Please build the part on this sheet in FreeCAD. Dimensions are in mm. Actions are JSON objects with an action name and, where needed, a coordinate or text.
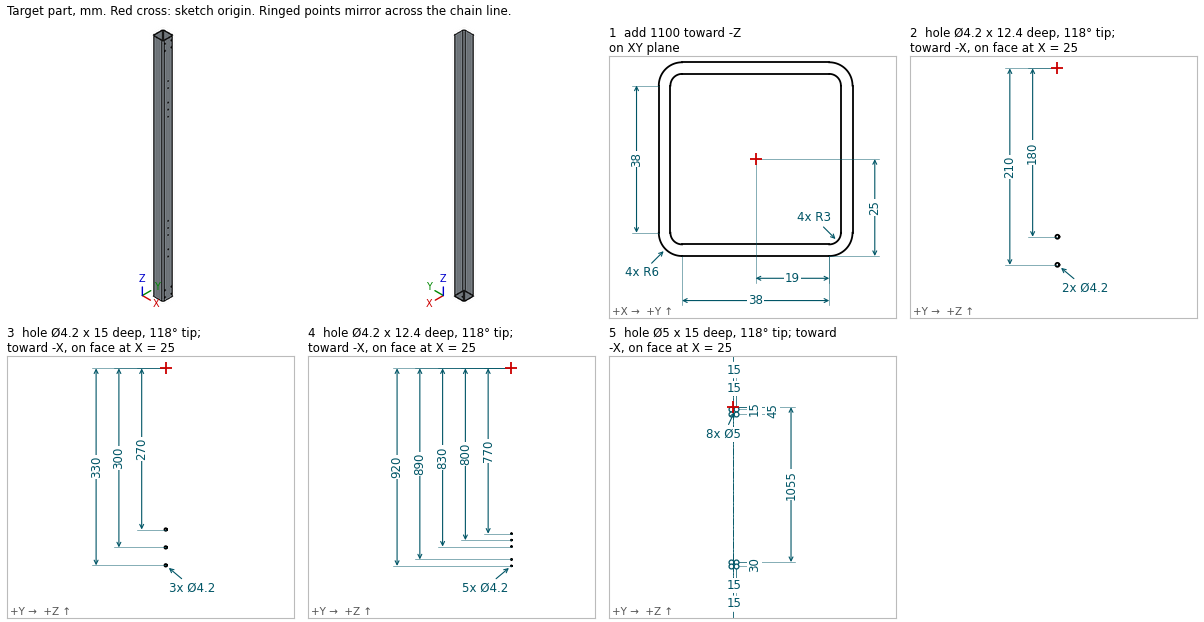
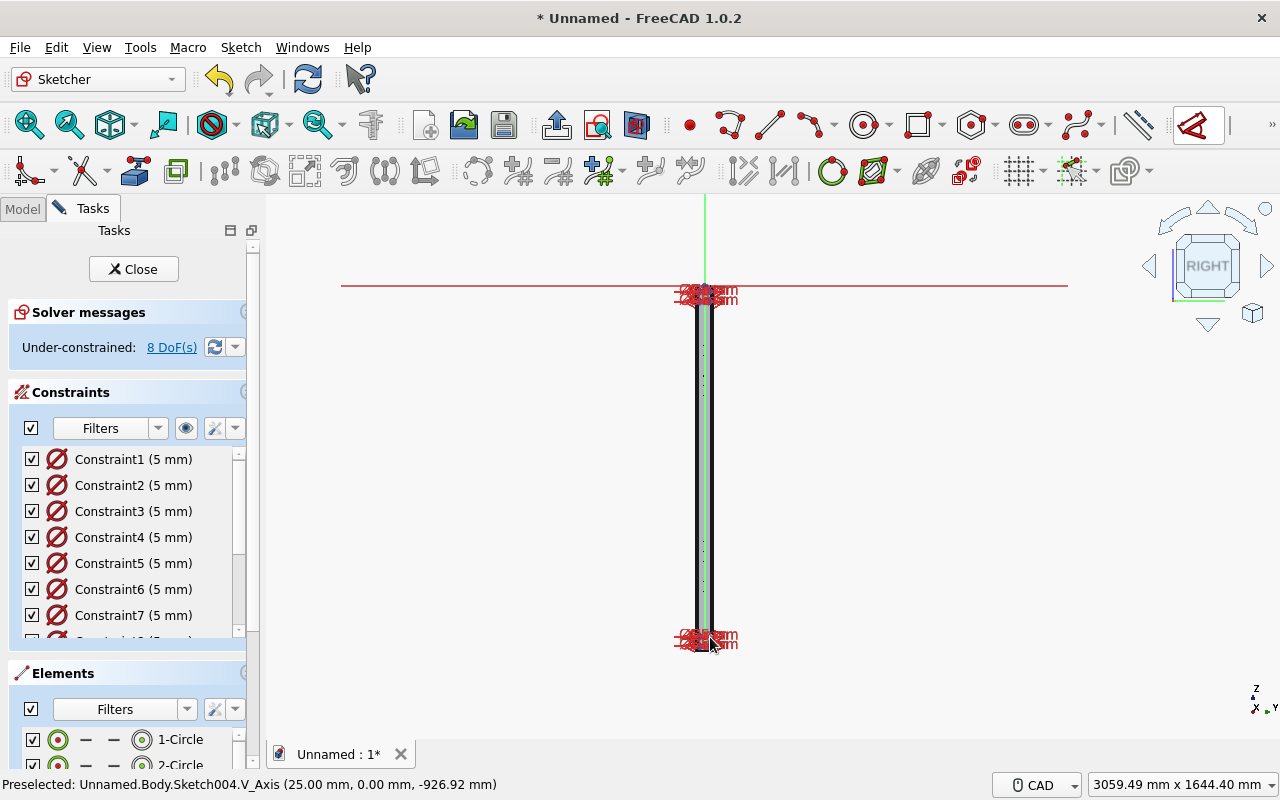
{"action": "scroll", "coordinate": [710, 292], "scroll_direction": "up", "scroll_amount": 11}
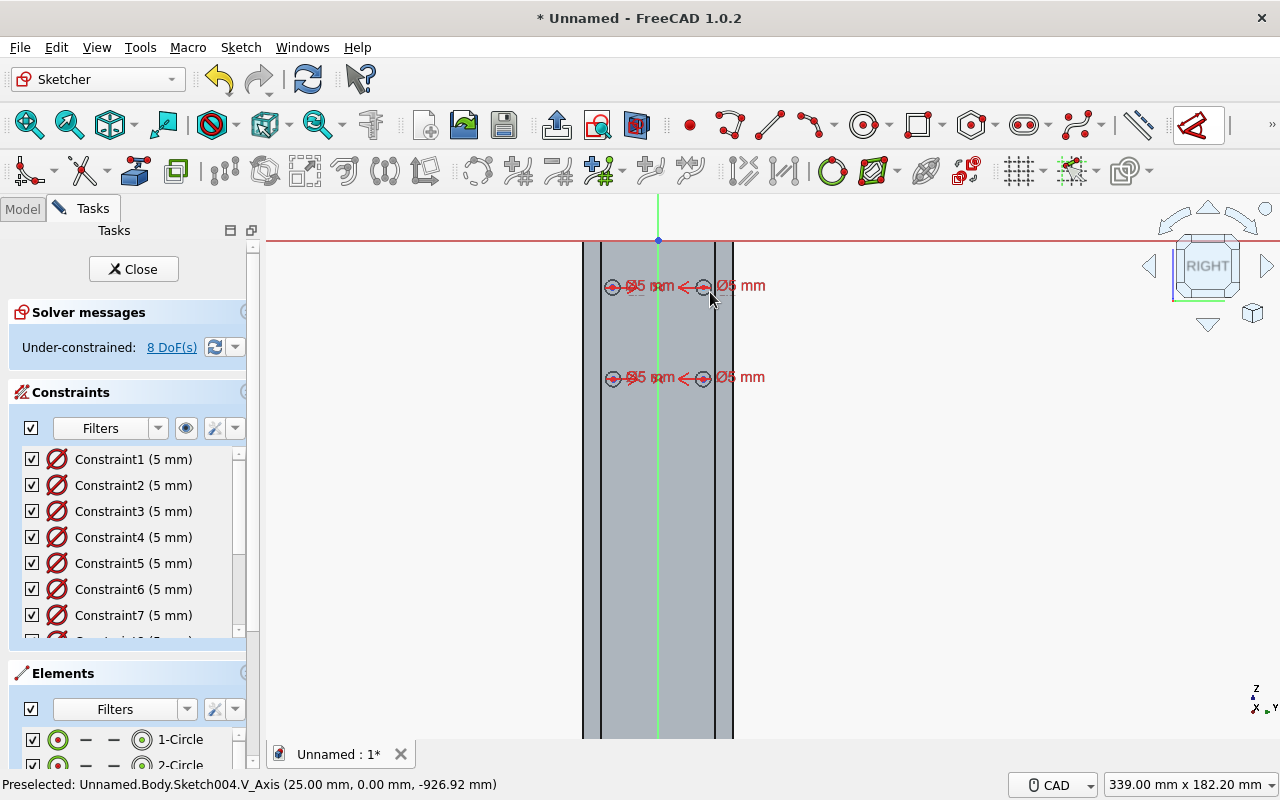
{"action": "left_click", "coordinate": [704, 288]}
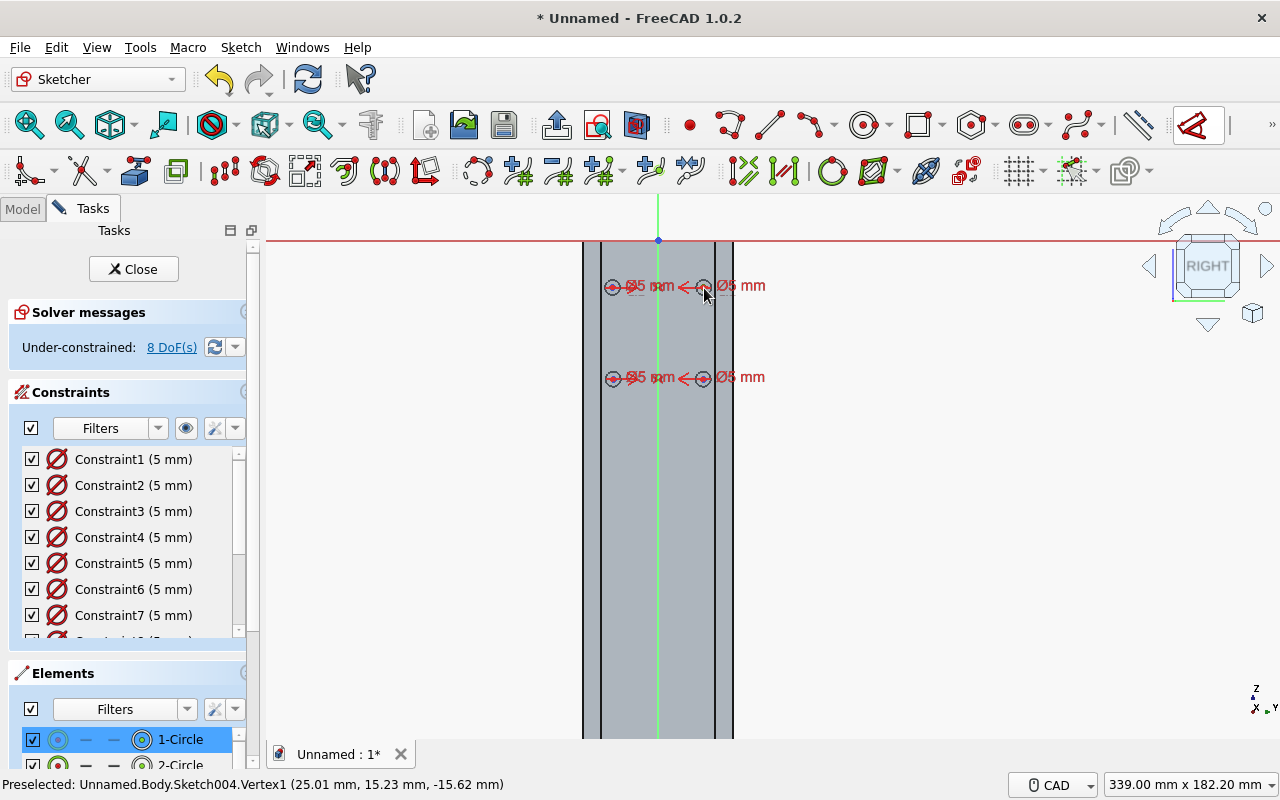
{"action": "left_click", "coordinate": [1218, 126]}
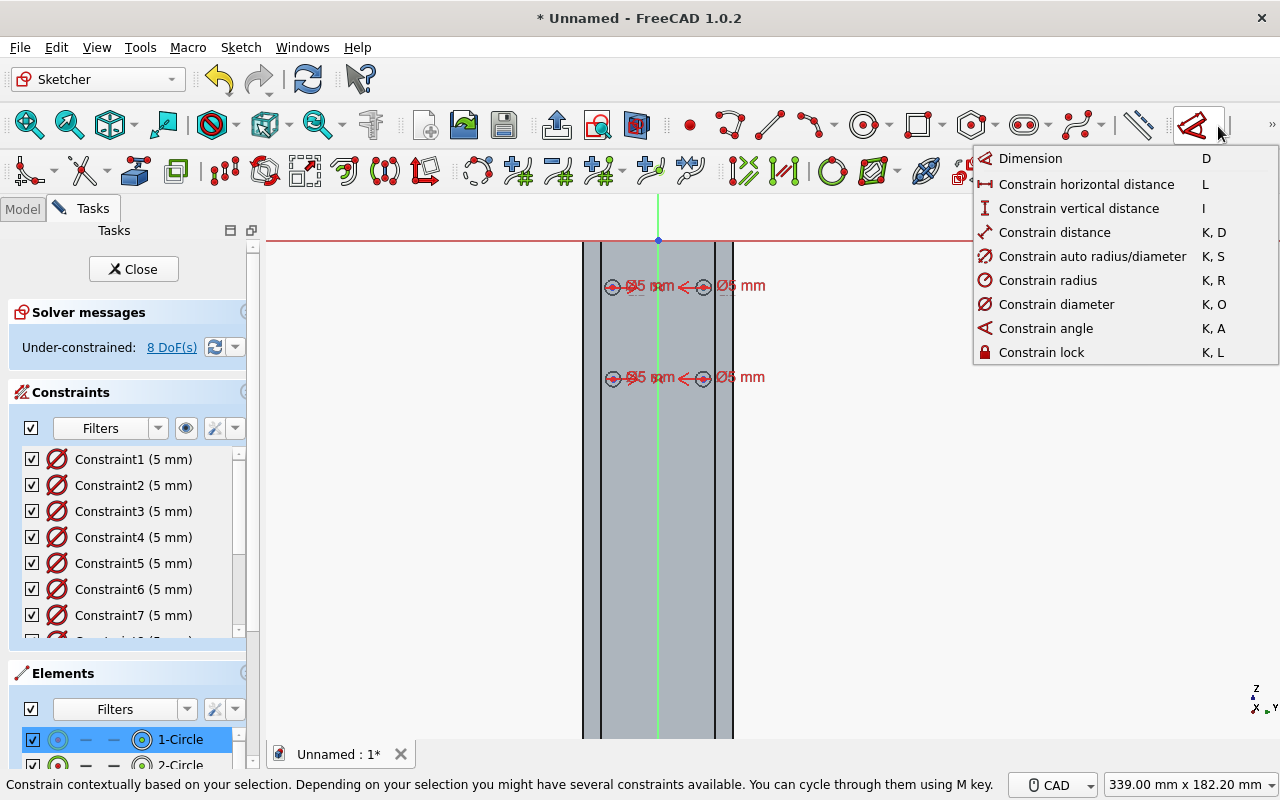
{"action": "left_click", "coordinate": [1126, 184]}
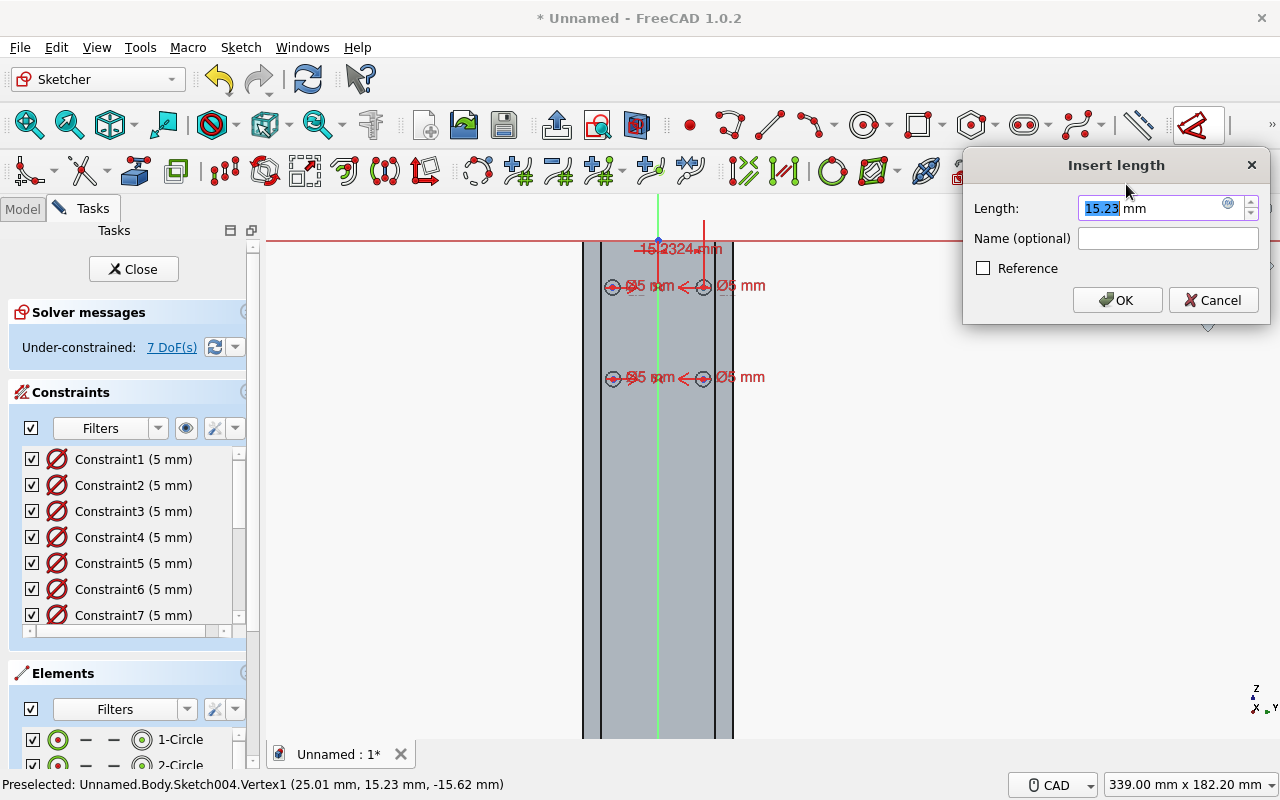
{"action": "type", "text": "15"}
{"action": "key", "text": "Return"}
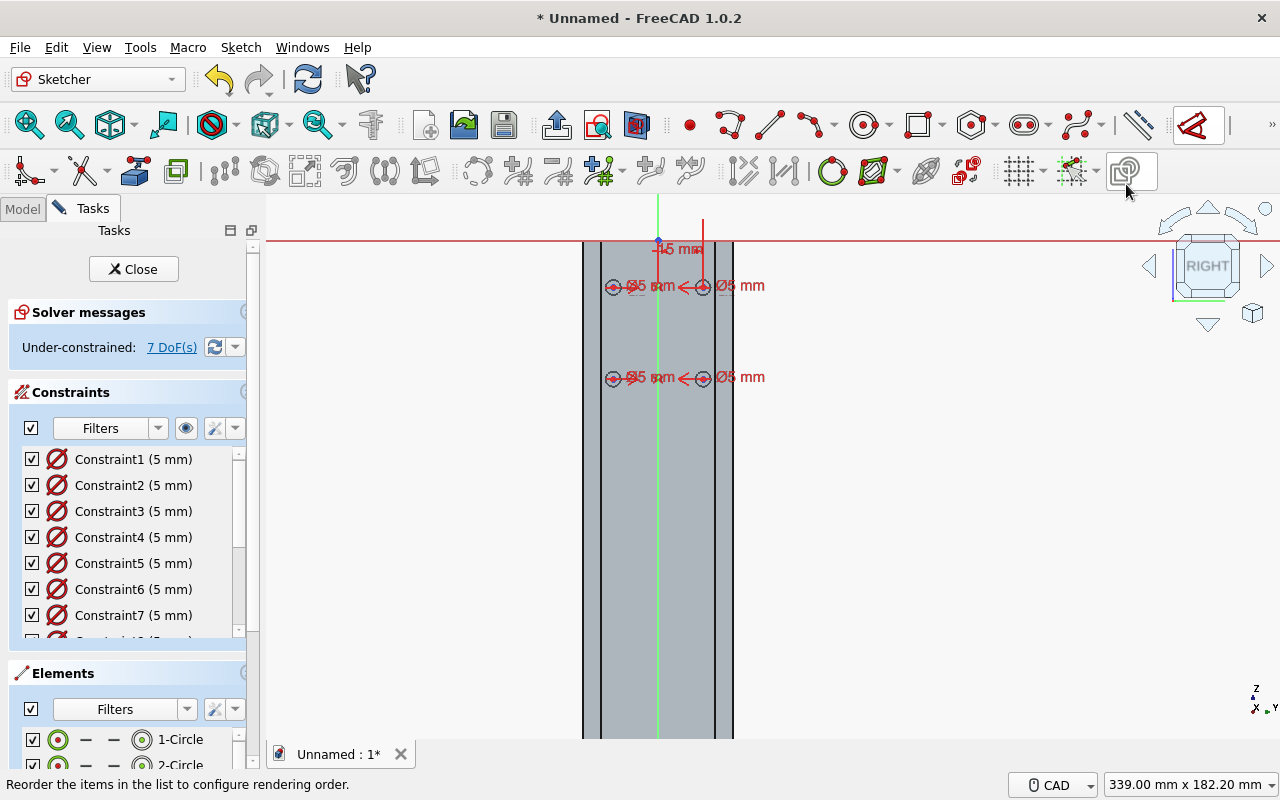
{"action": "left_click", "coordinate": [703, 288]}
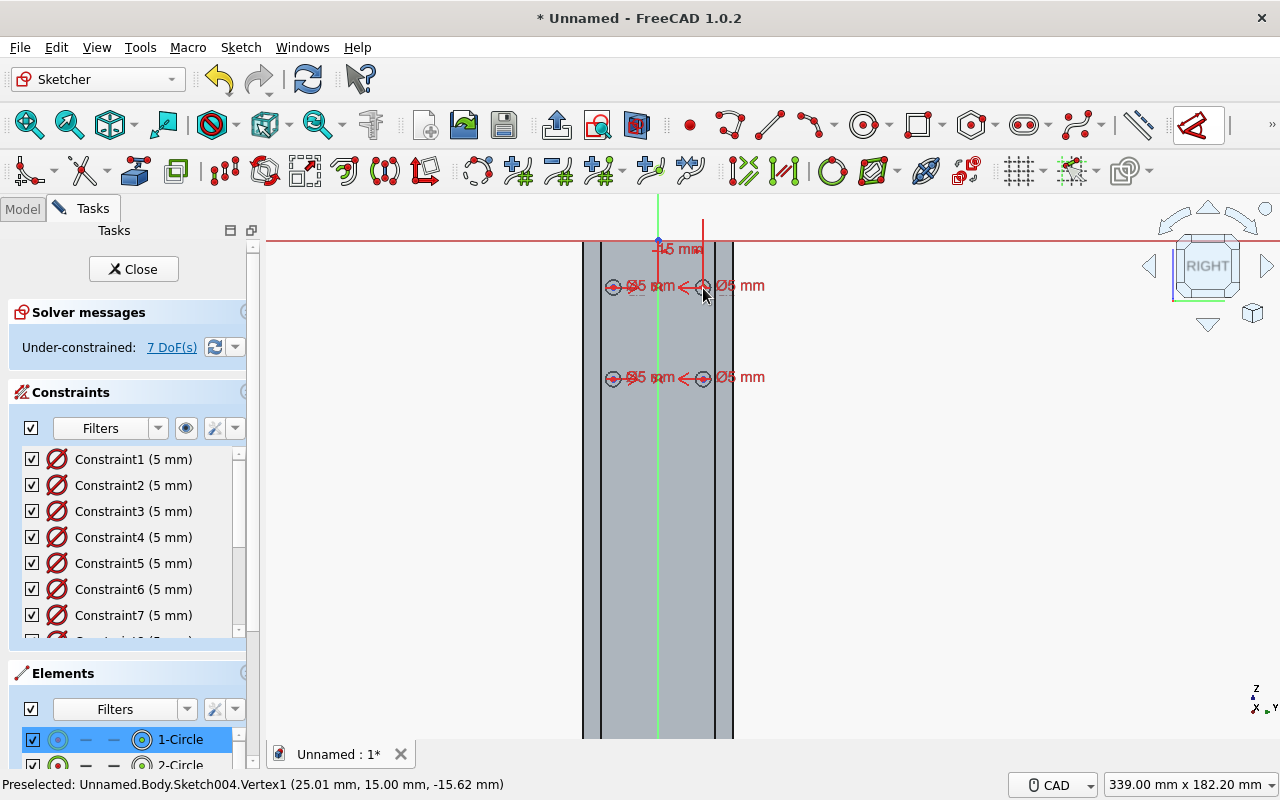
{"action": "left_click", "coordinate": [1218, 126]}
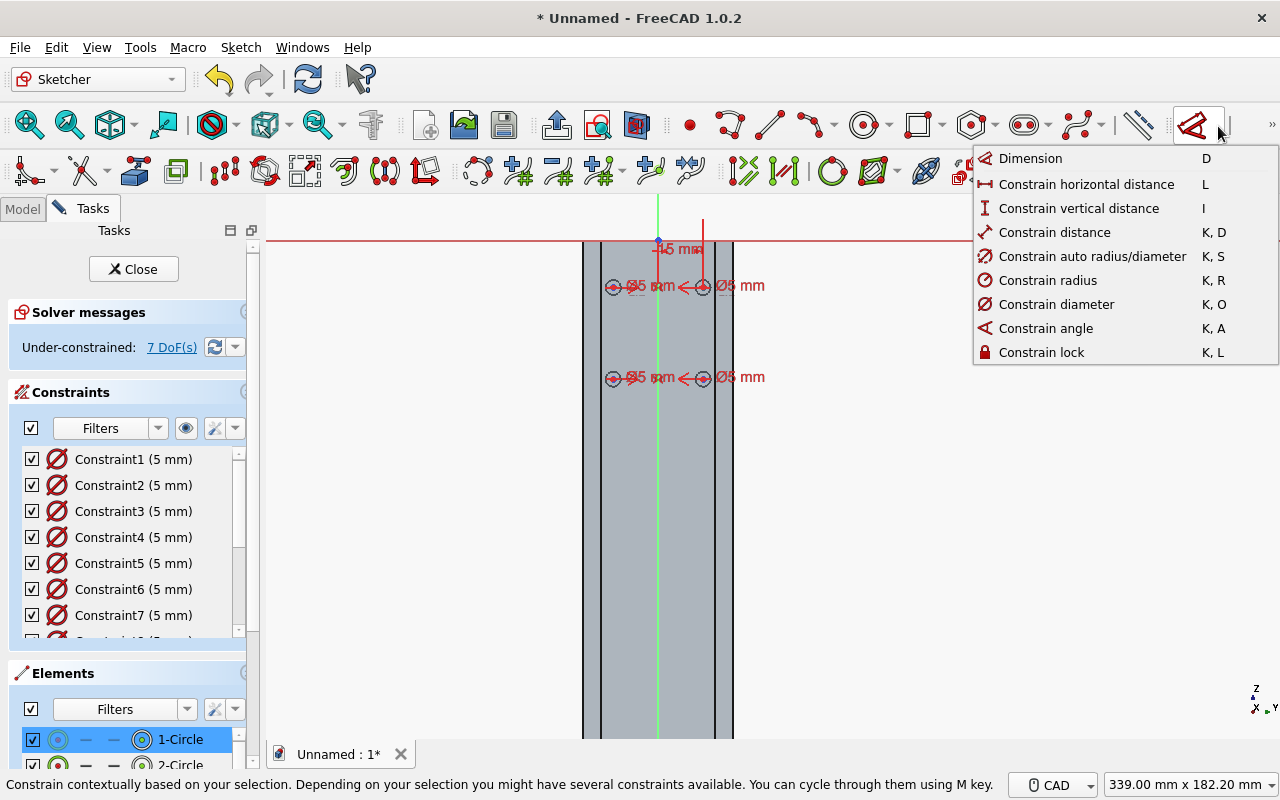
{"action": "left_click", "coordinate": [1126, 208]}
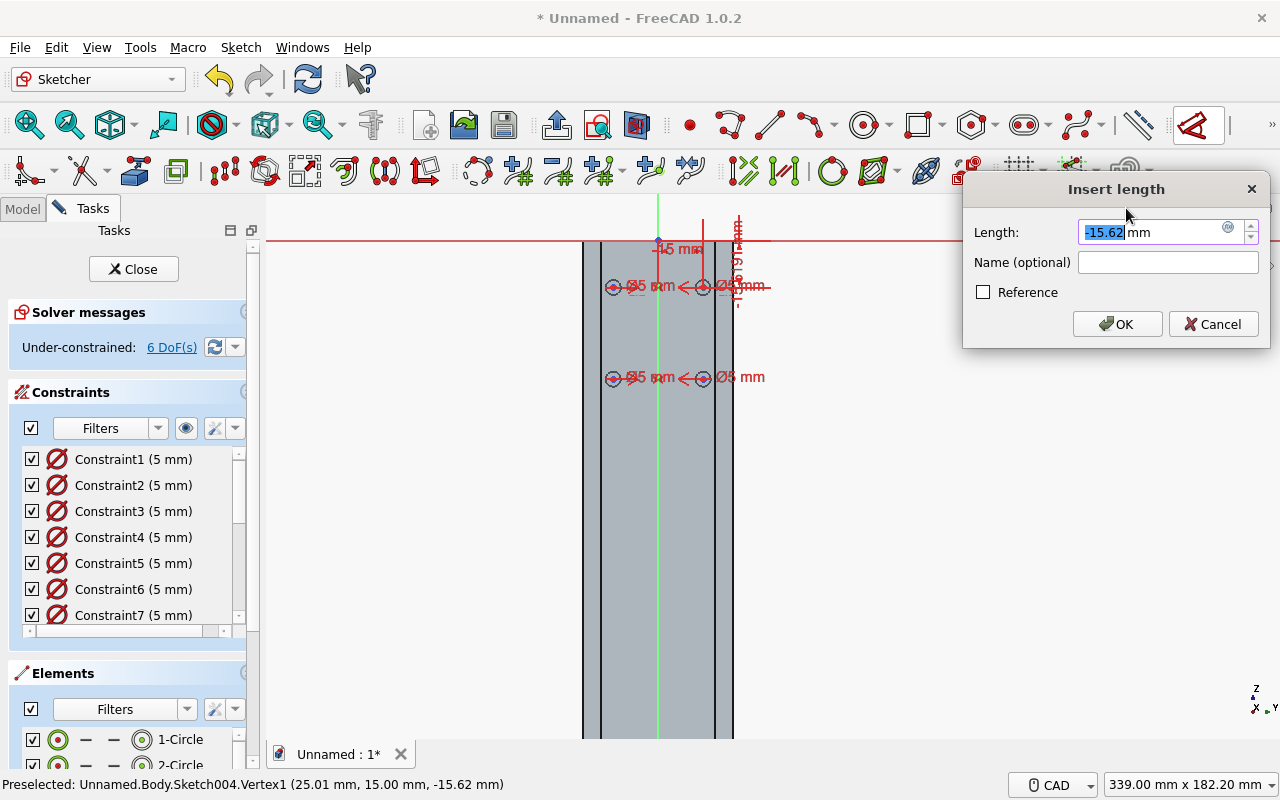
{"action": "type", "text": "-15"}
{"action": "key", "text": "Return"}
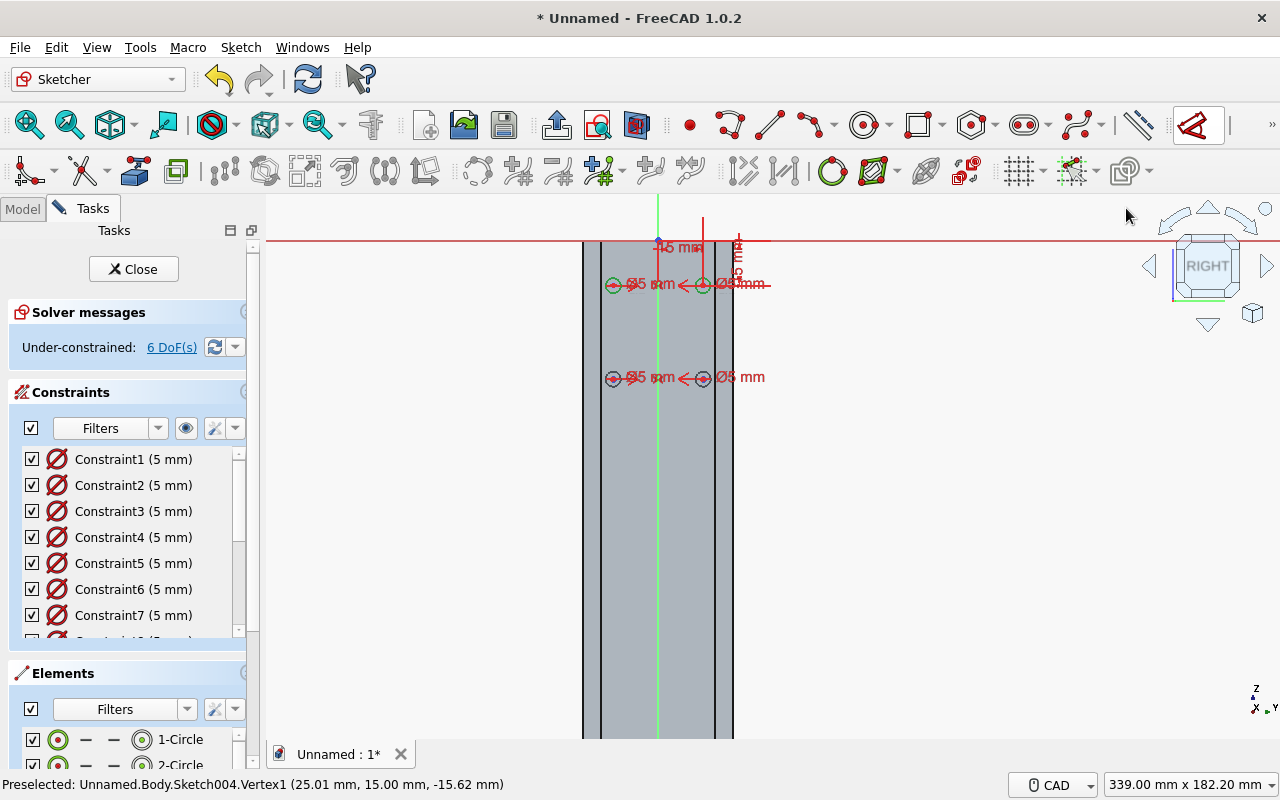
{"action": "left_click", "coordinate": [703, 379]}